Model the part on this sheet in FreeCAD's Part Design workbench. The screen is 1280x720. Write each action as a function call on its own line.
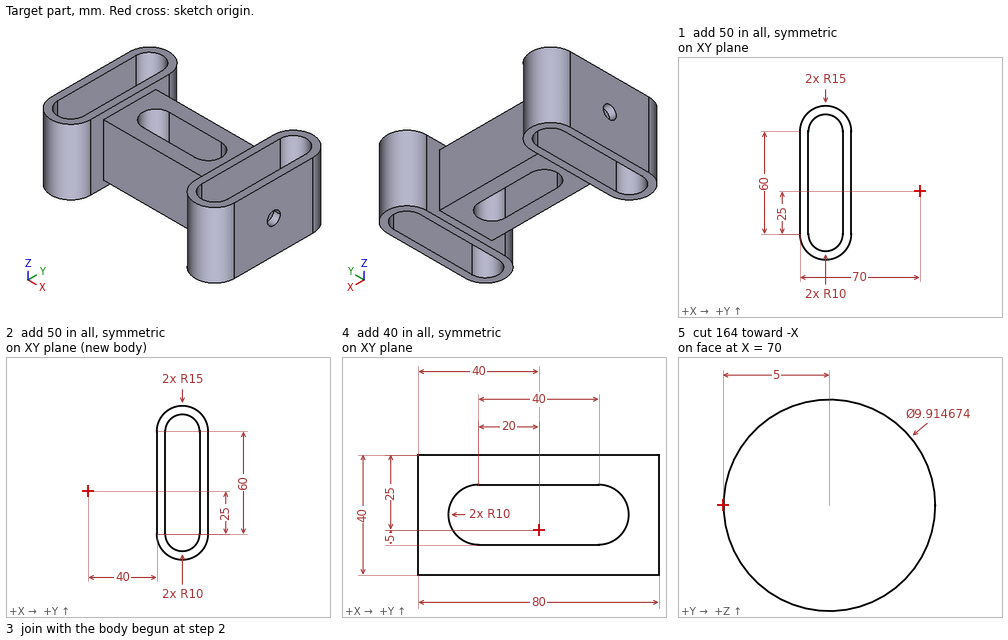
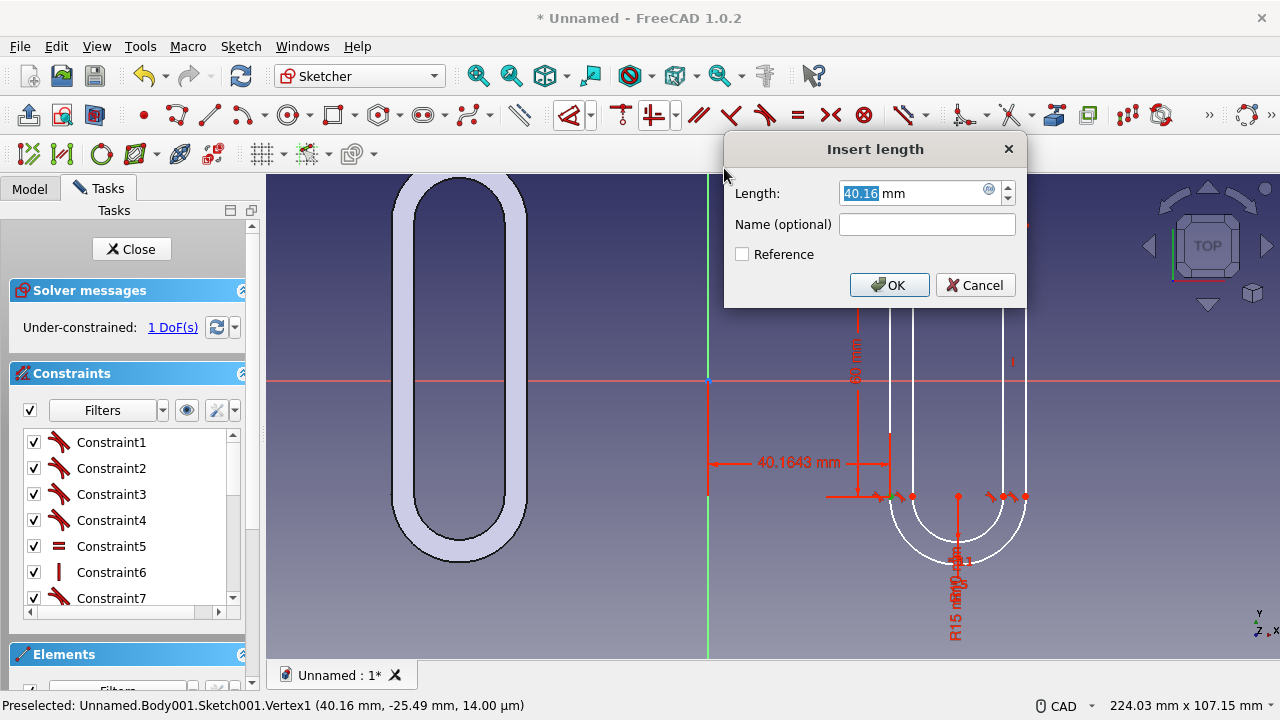
text(40)
key(Return)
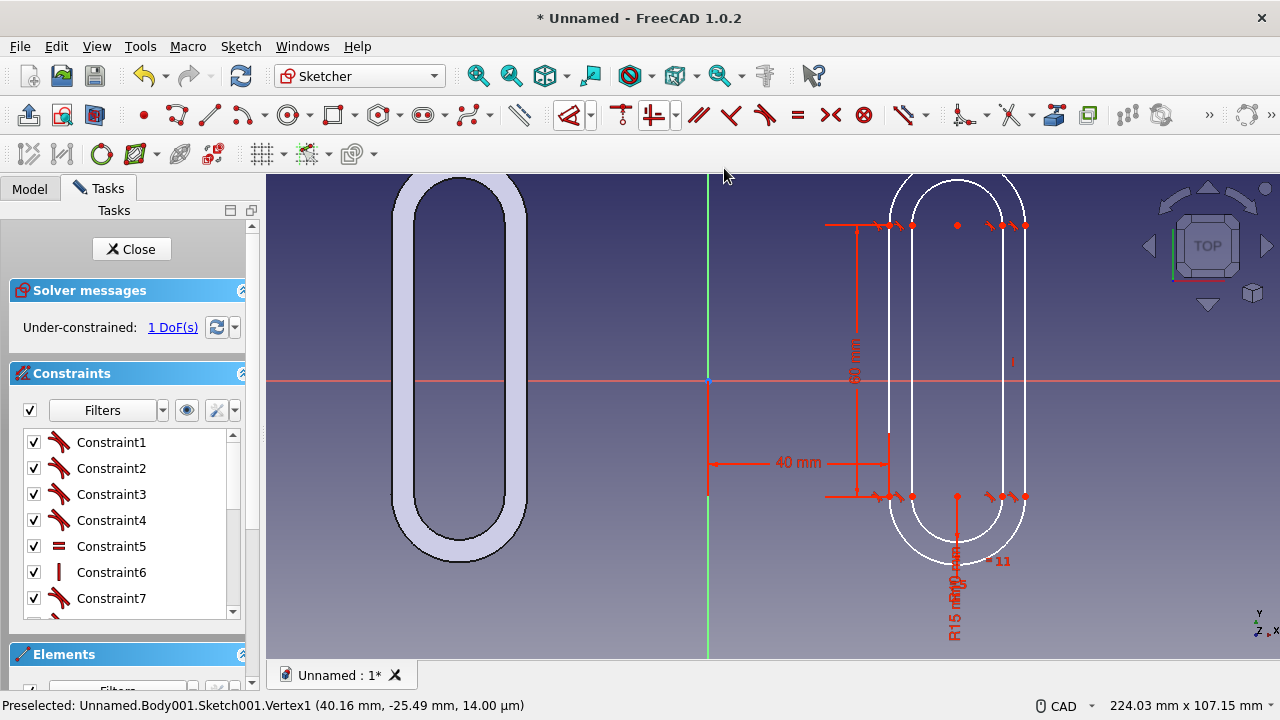
click(889, 497)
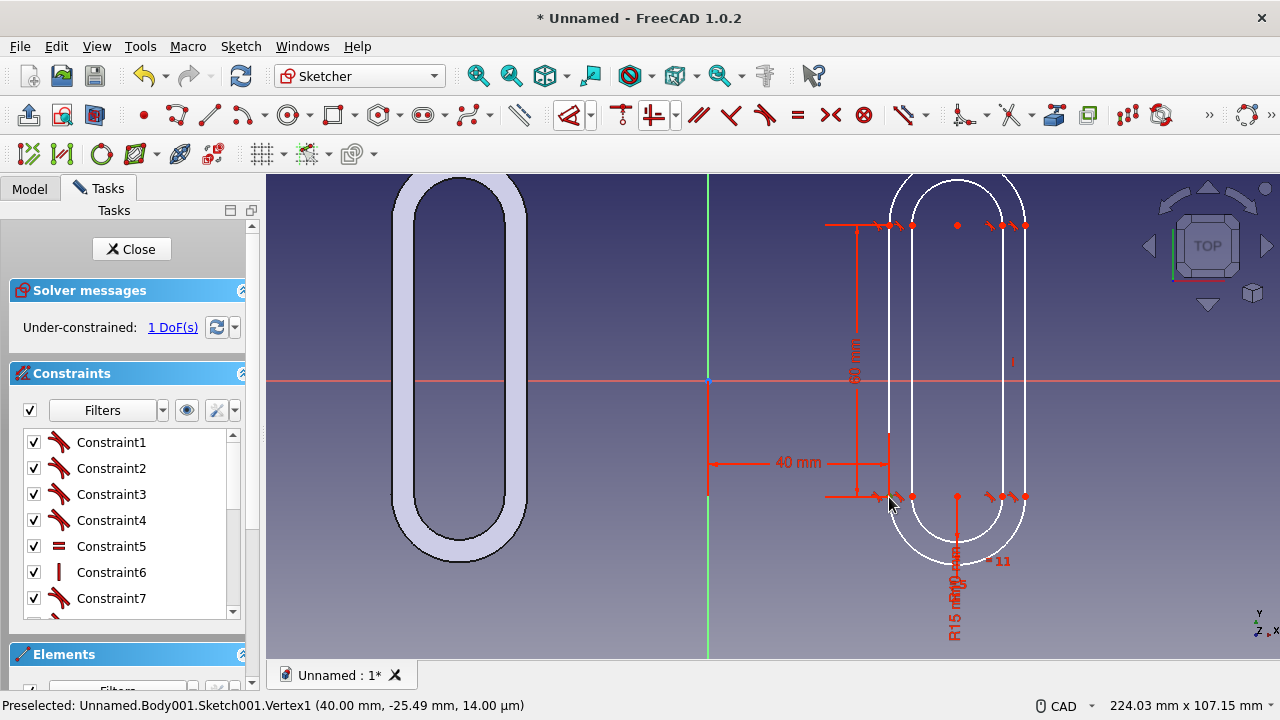
click(590, 116)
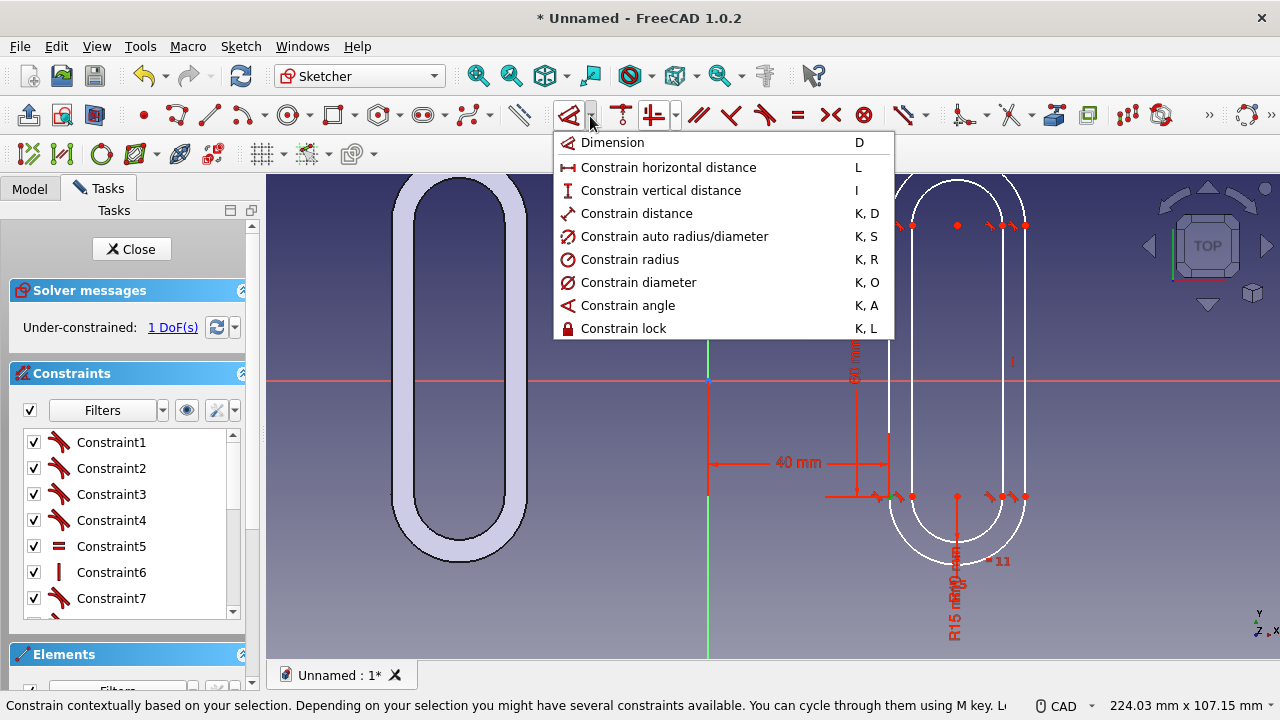
click(724, 190)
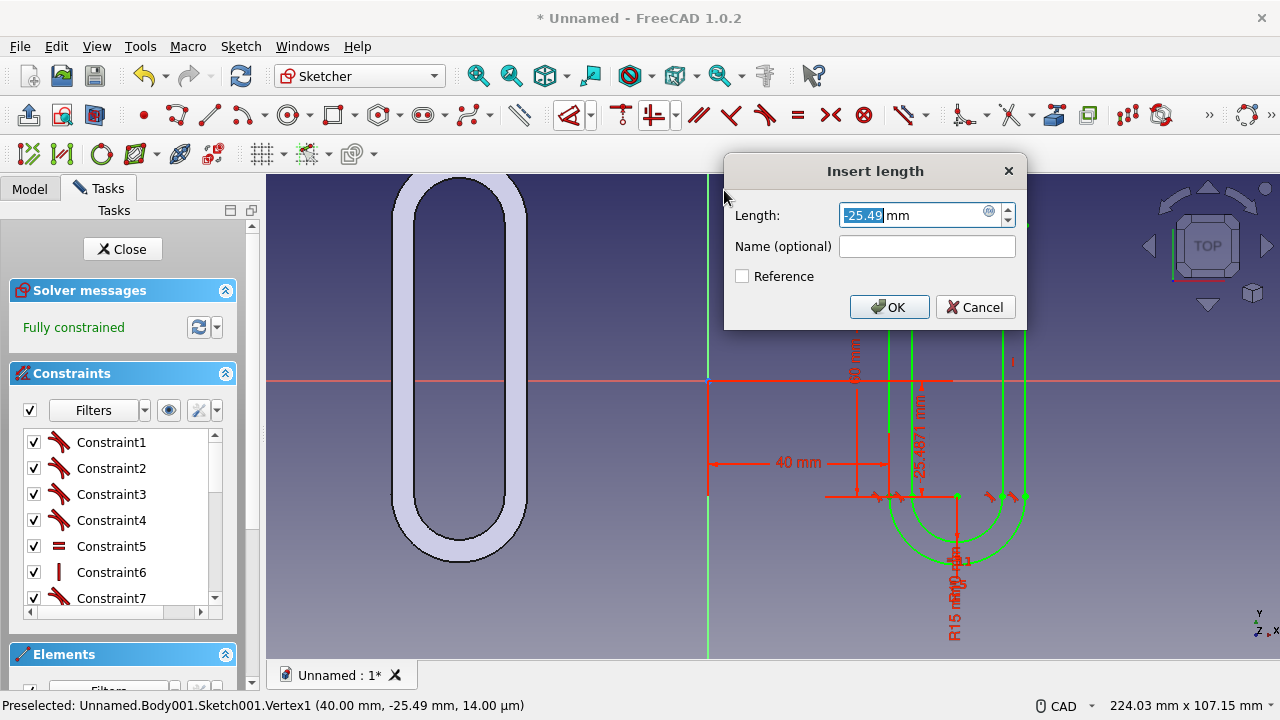
text(-25)
key(Return)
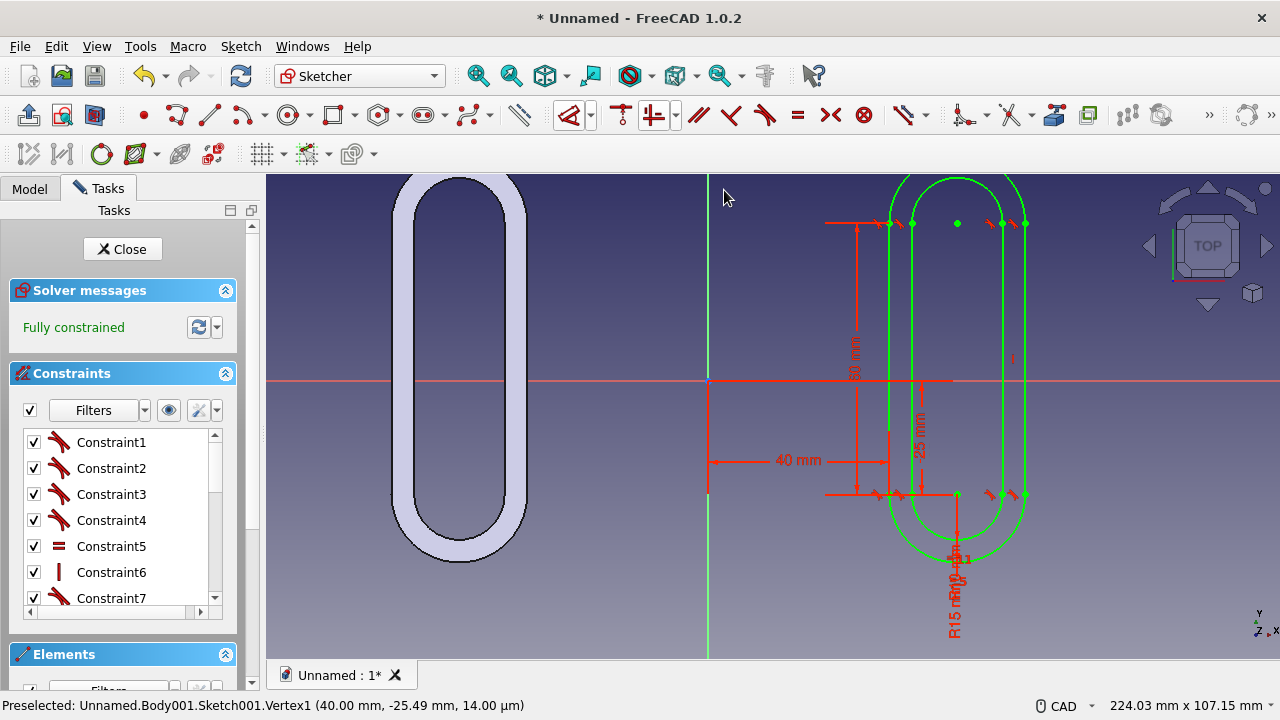
click(123, 249)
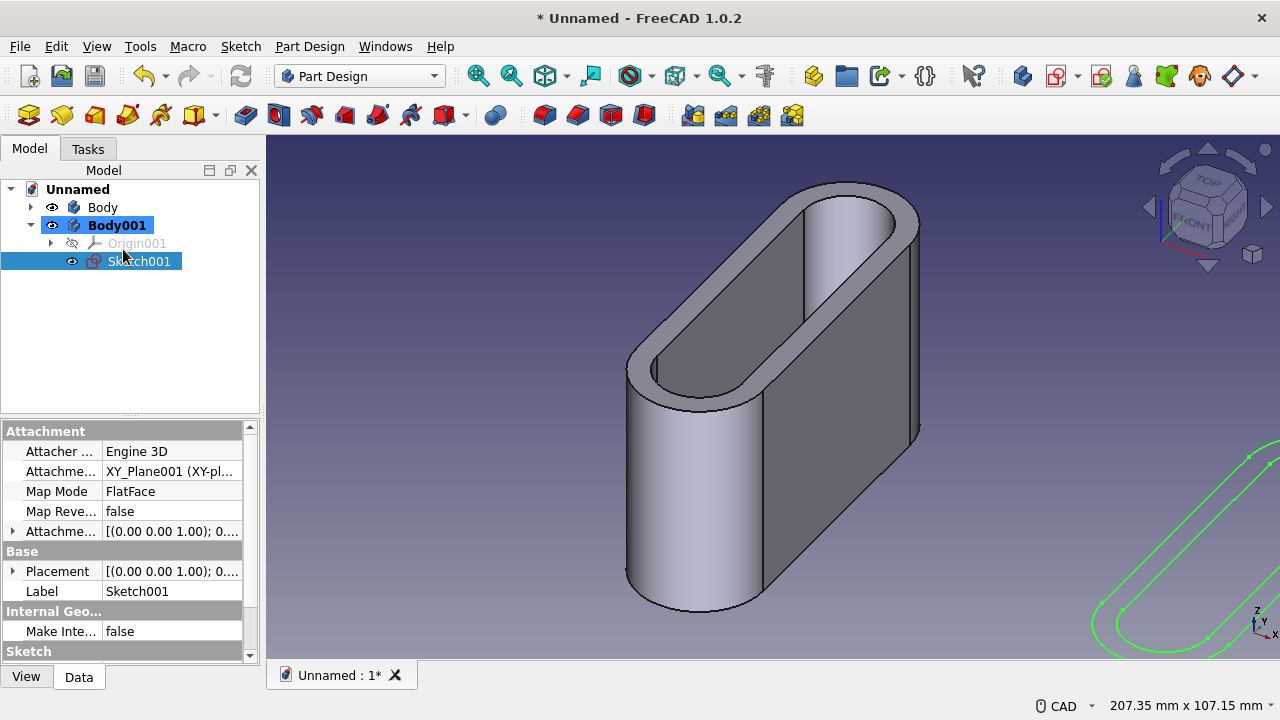
click(29, 116)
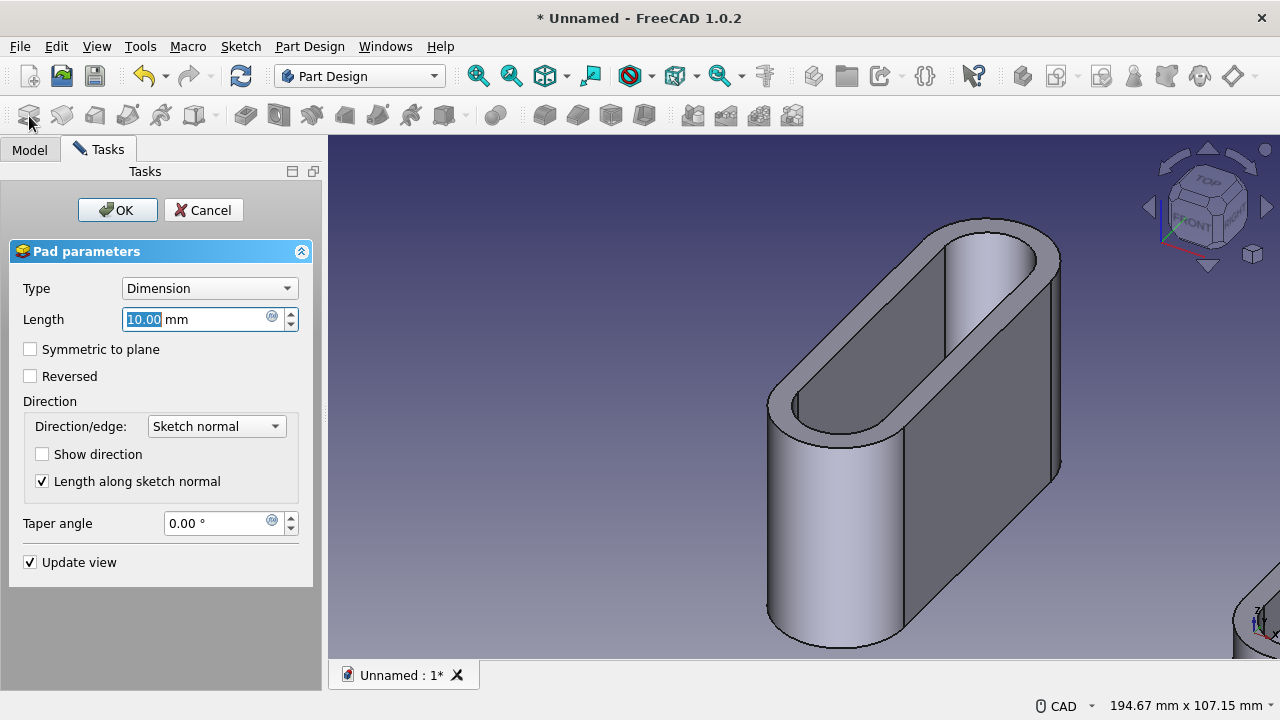
text(50)
key(Tab)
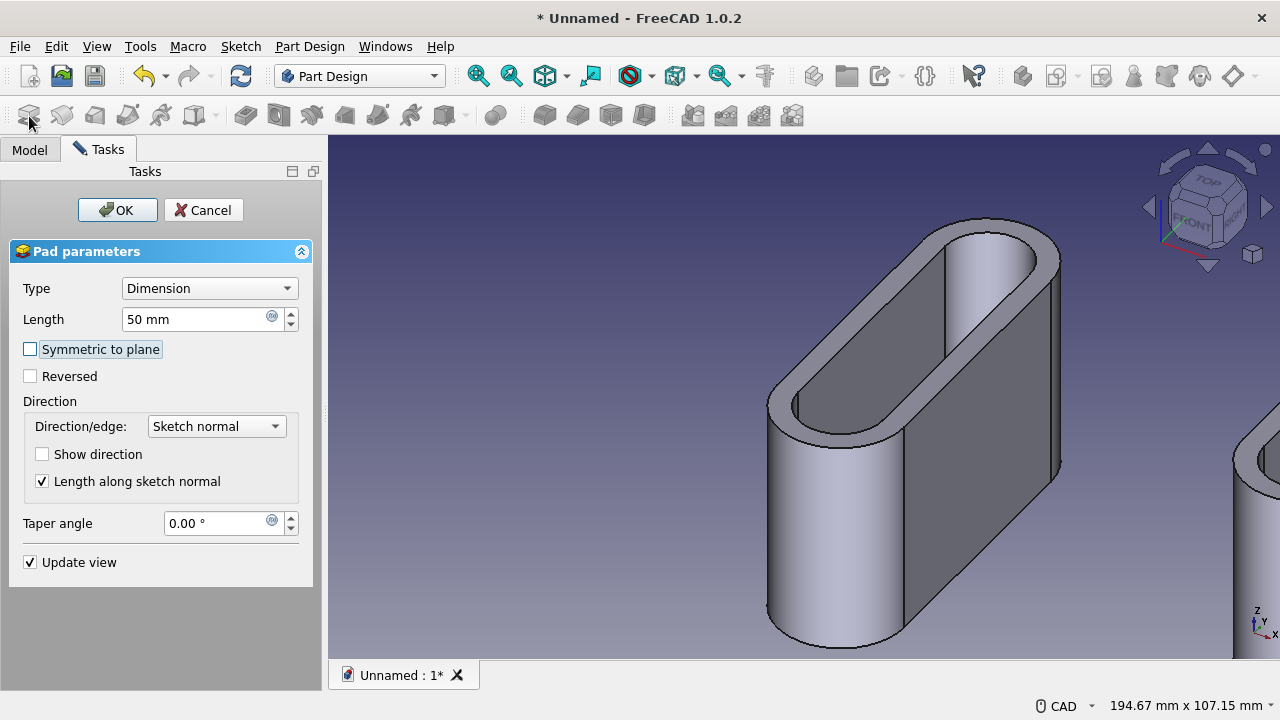
click(31, 349)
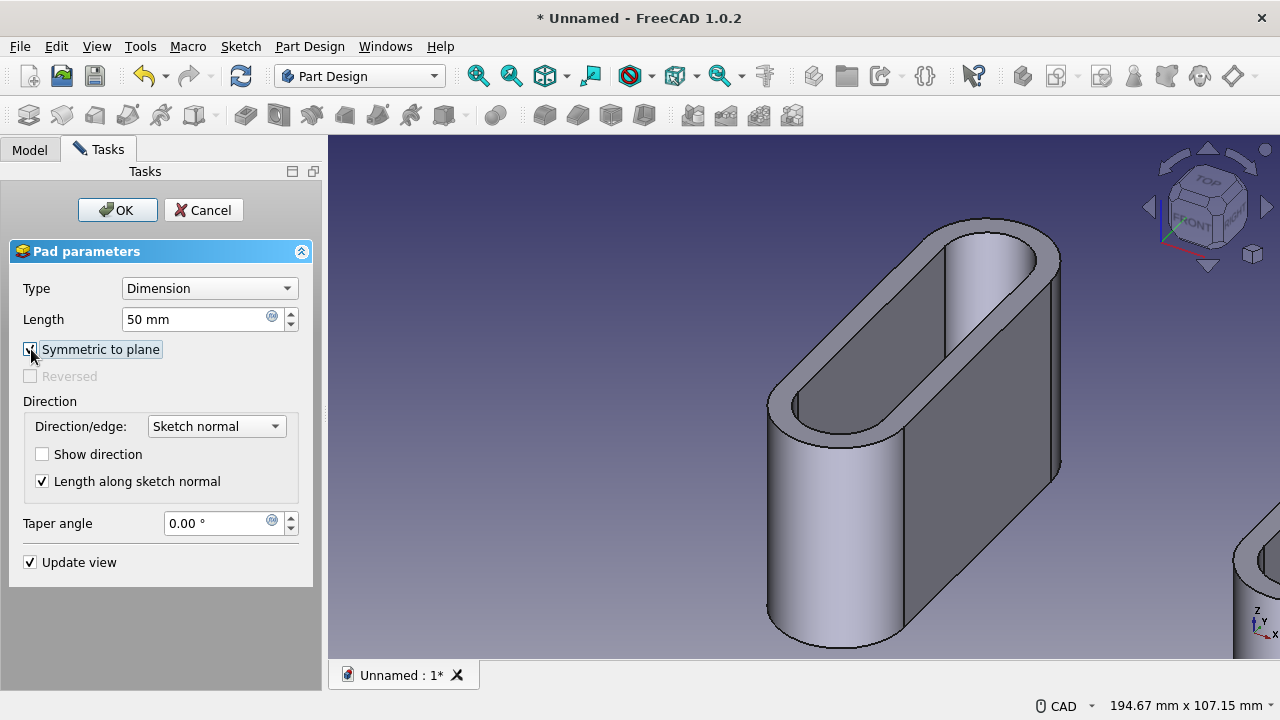
click(118, 210)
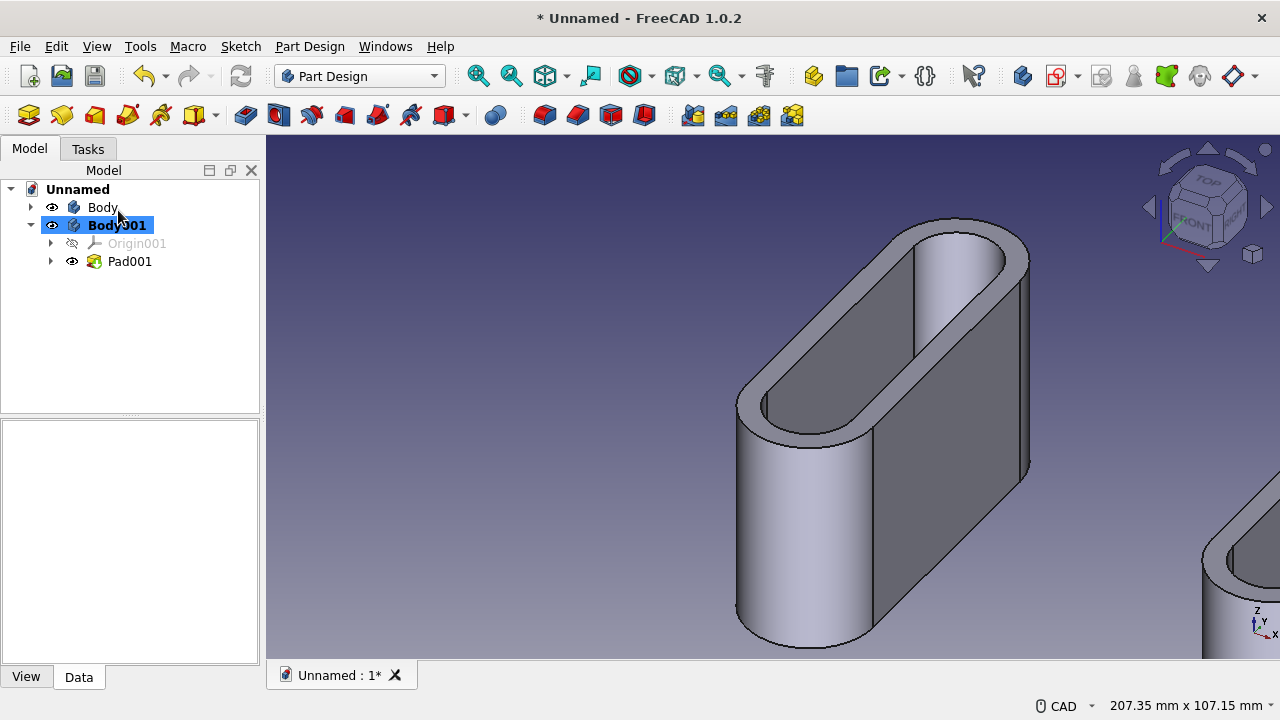
click(479, 76)